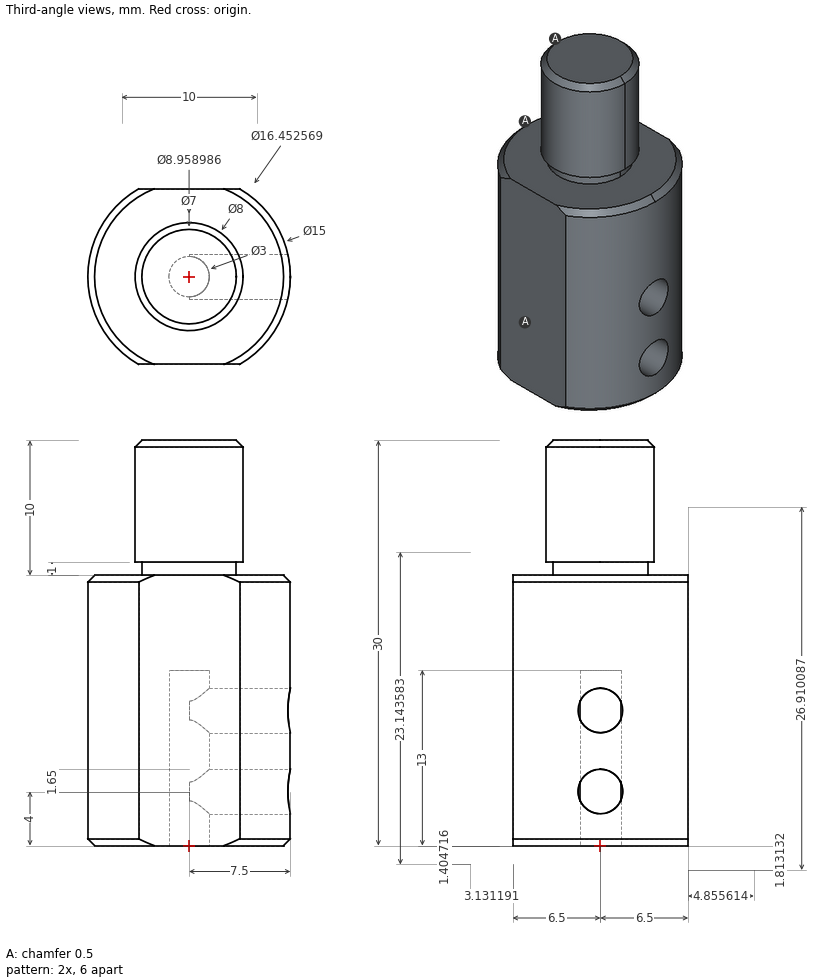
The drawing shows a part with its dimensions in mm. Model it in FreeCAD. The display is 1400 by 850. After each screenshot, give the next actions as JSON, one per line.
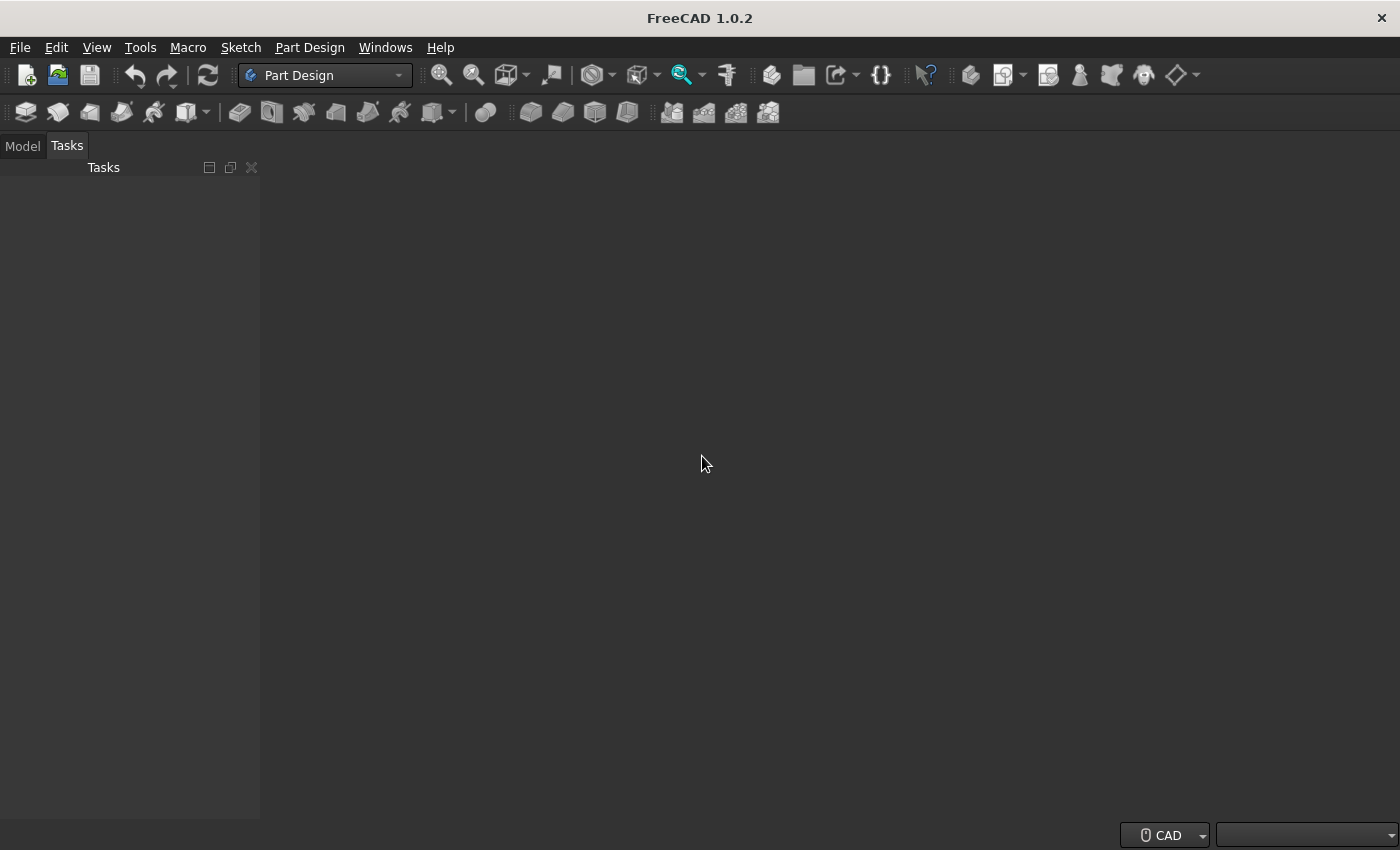
{"action": "left_click", "coordinate": [26, 76]}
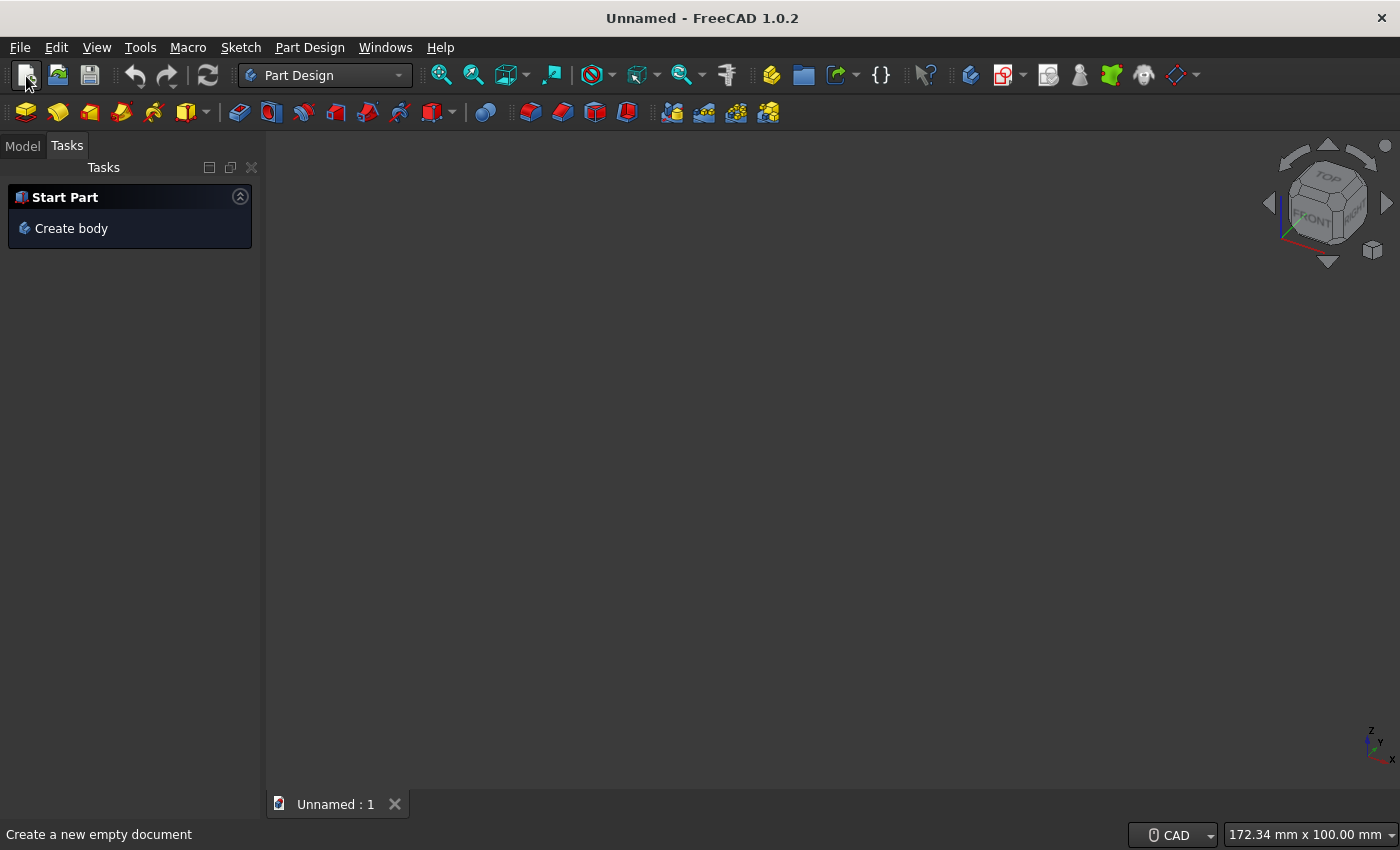
{"action": "left_click", "coordinate": [1004, 76]}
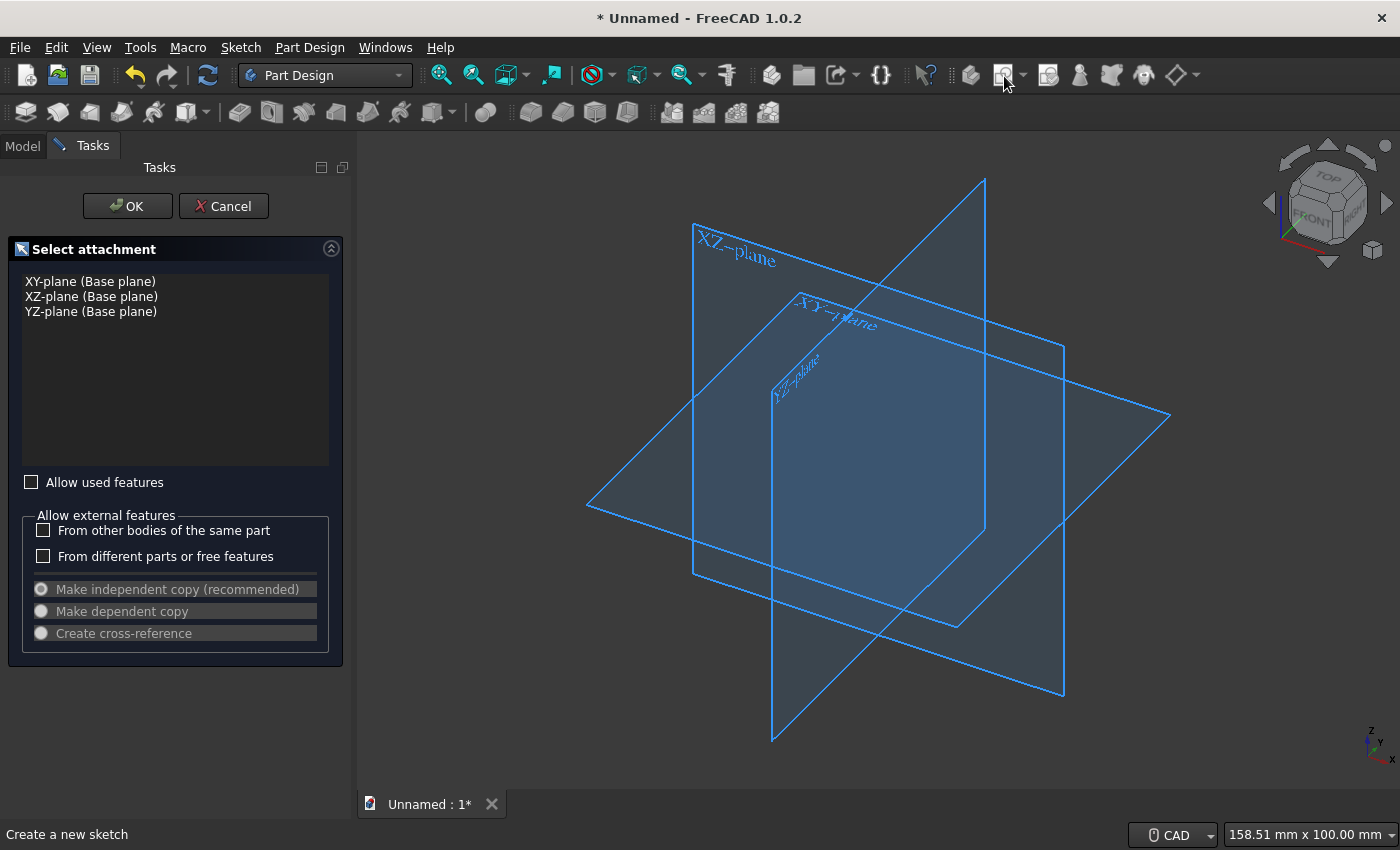
{"action": "left_click", "coordinate": [82, 282]}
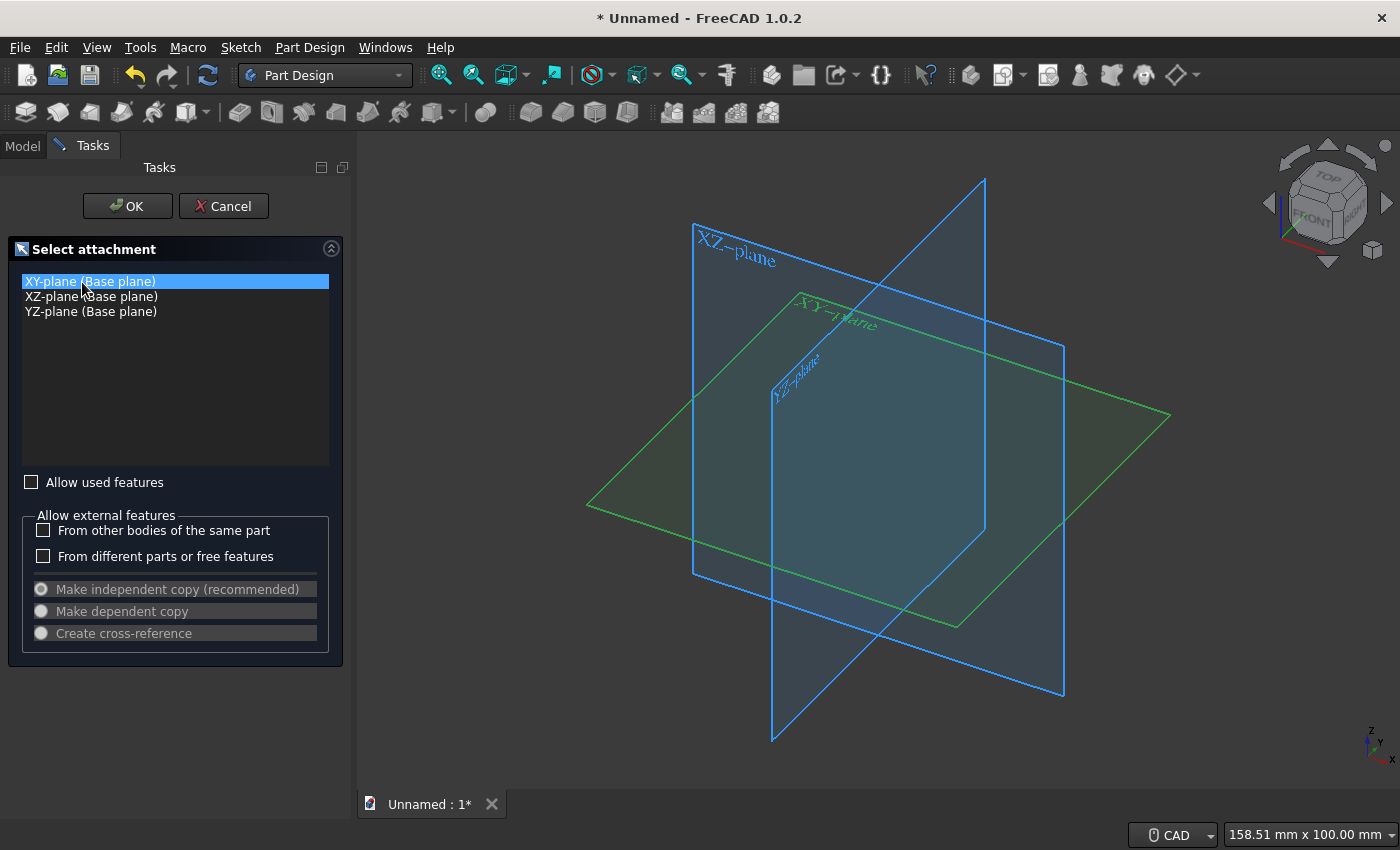
{"action": "left_click", "coordinate": [128, 206]}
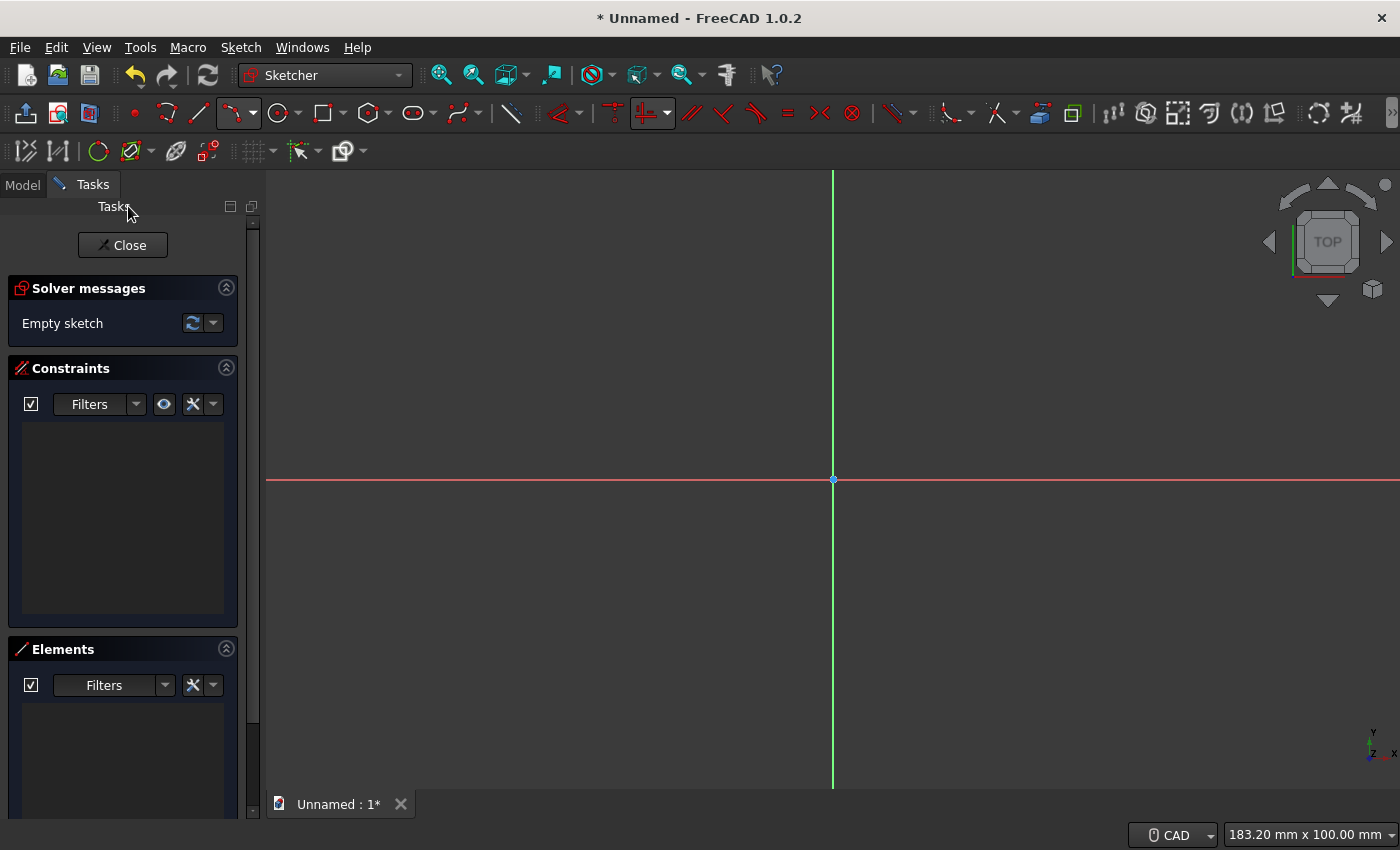
{"action": "scroll", "coordinate": [855, 480], "scroll_direction": "up", "scroll_amount": 7}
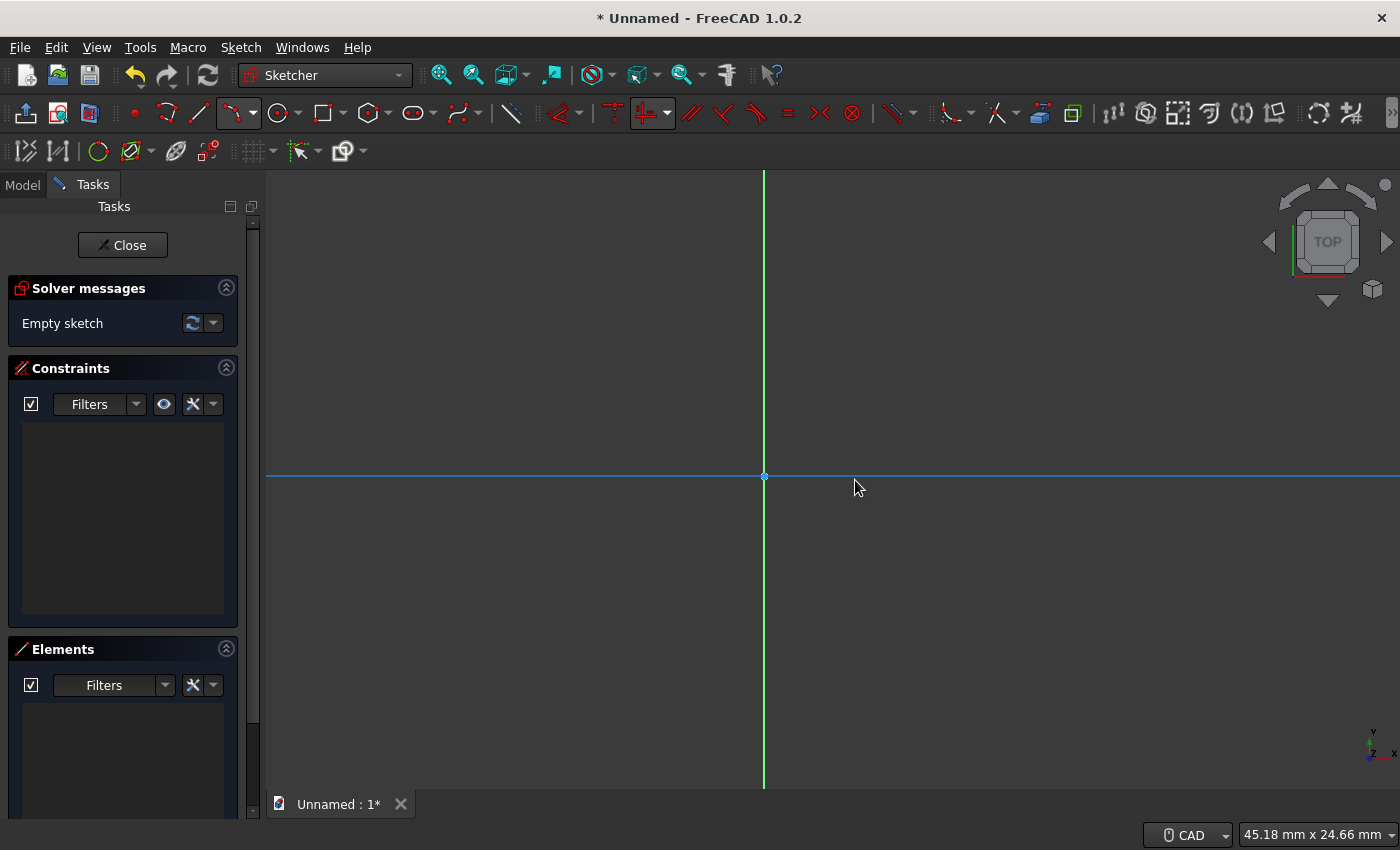
{"action": "left_click", "coordinate": [278, 114]}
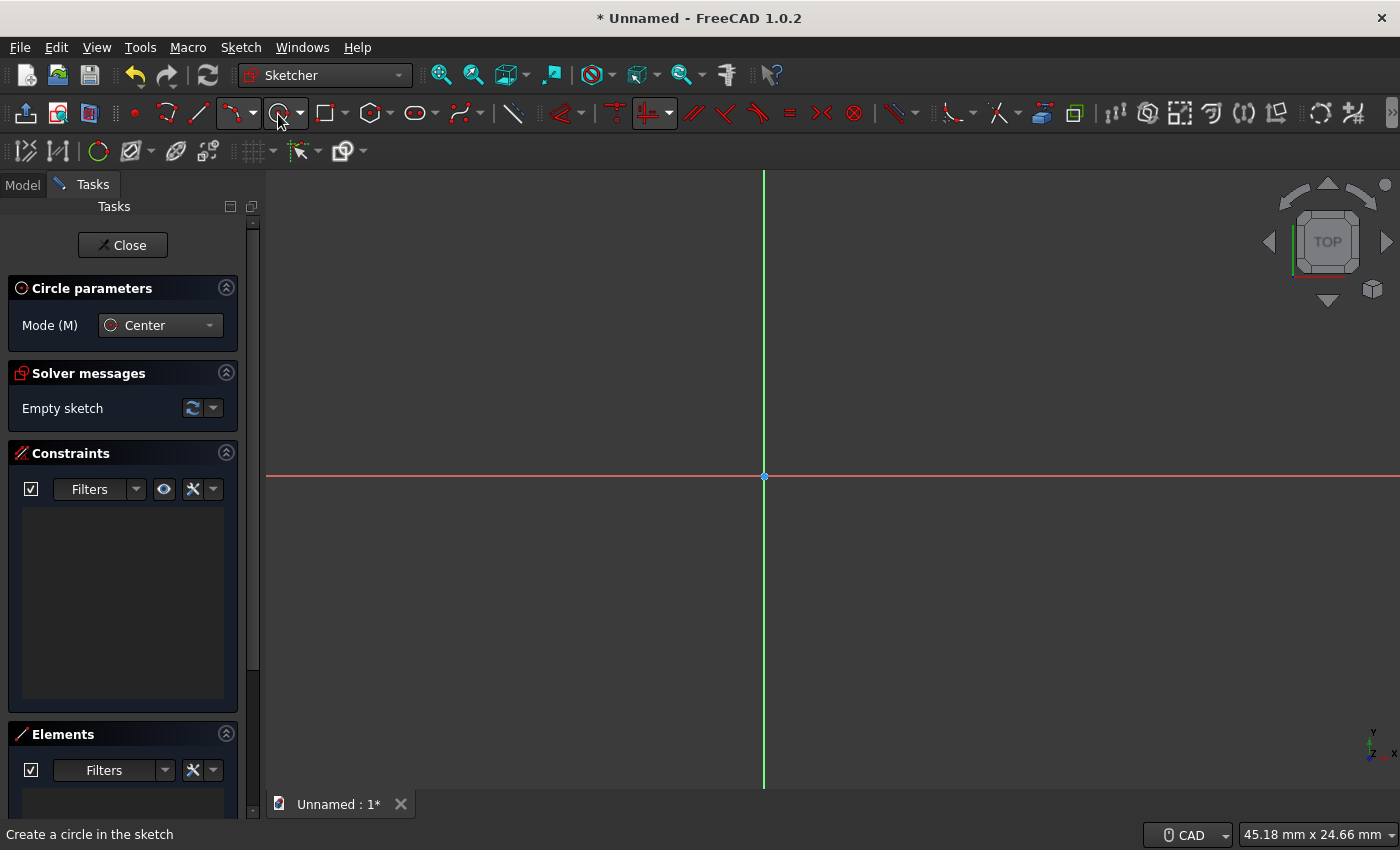
{"action": "left_click", "coordinate": [764, 476]}
{"action": "left_click", "coordinate": [897, 343]}
{"action": "key", "text": "Escape"}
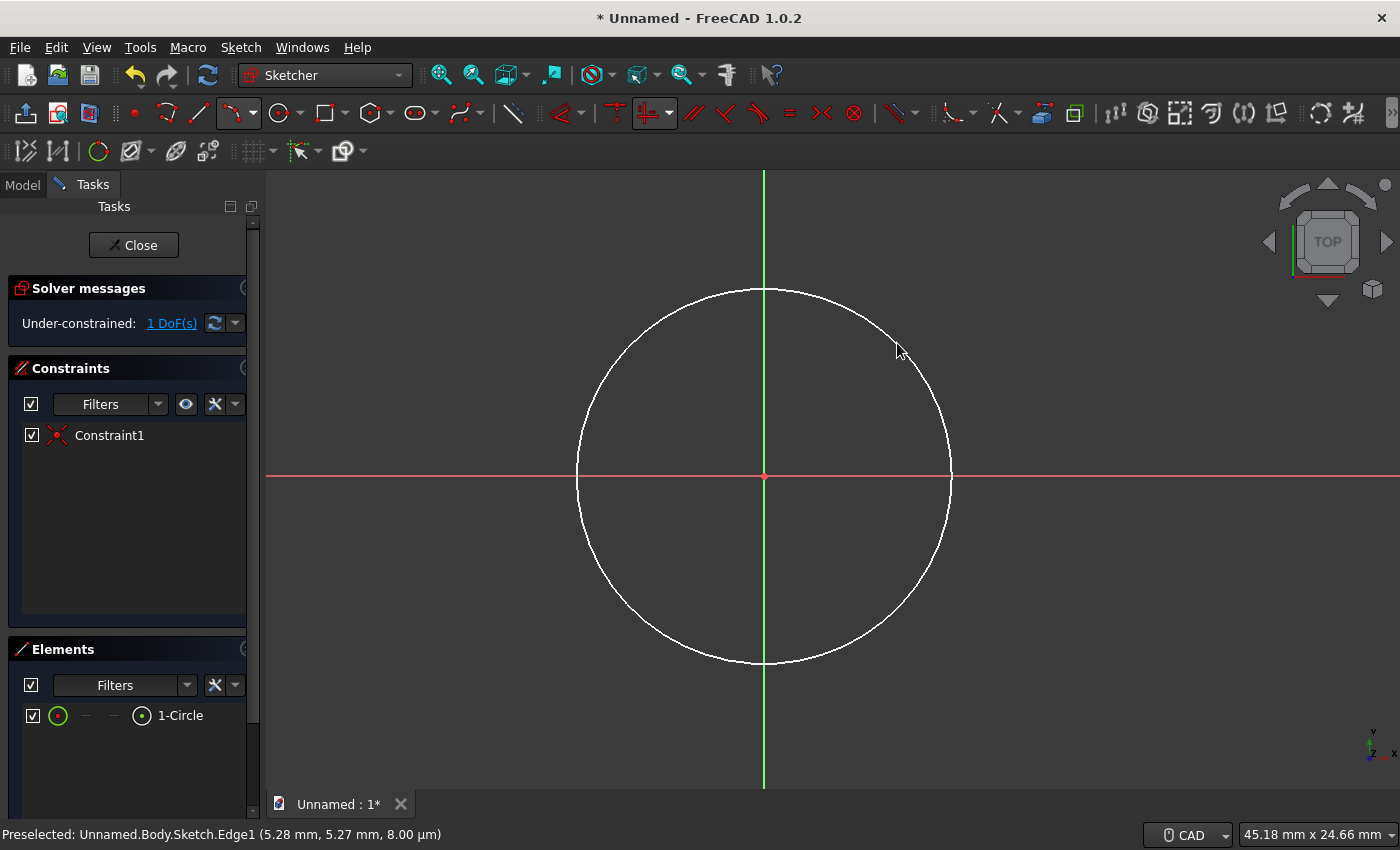
{"action": "left_click", "coordinate": [560, 114]}